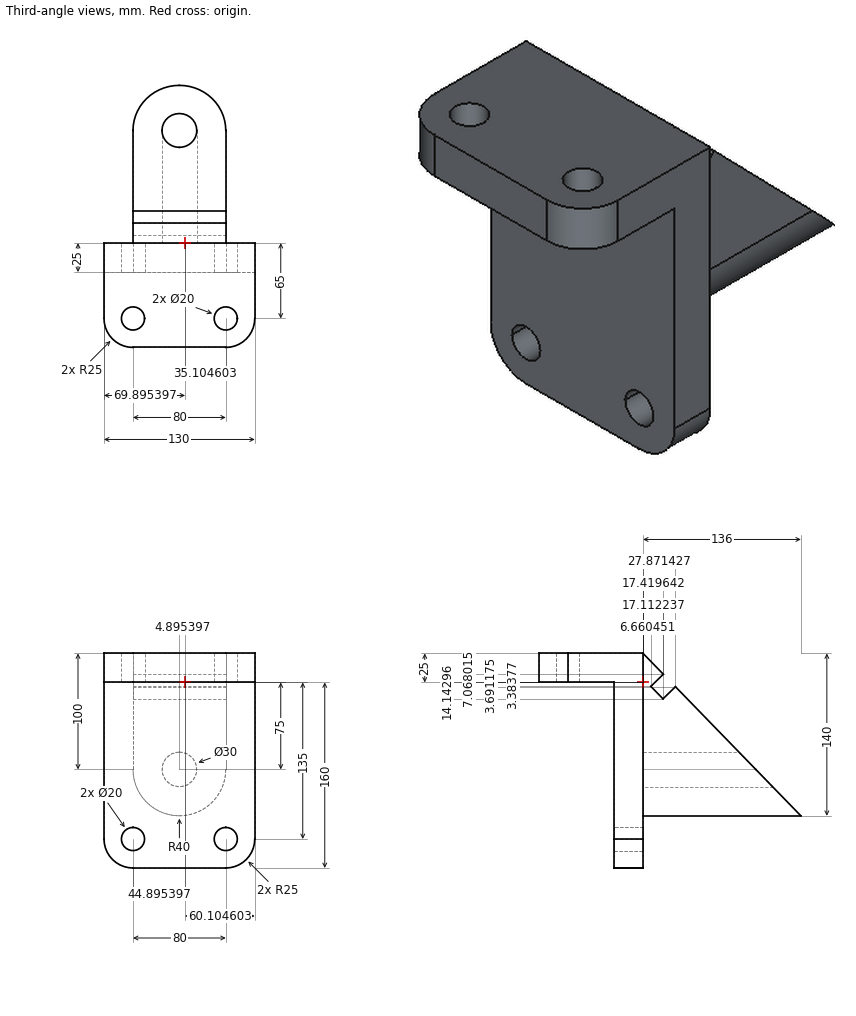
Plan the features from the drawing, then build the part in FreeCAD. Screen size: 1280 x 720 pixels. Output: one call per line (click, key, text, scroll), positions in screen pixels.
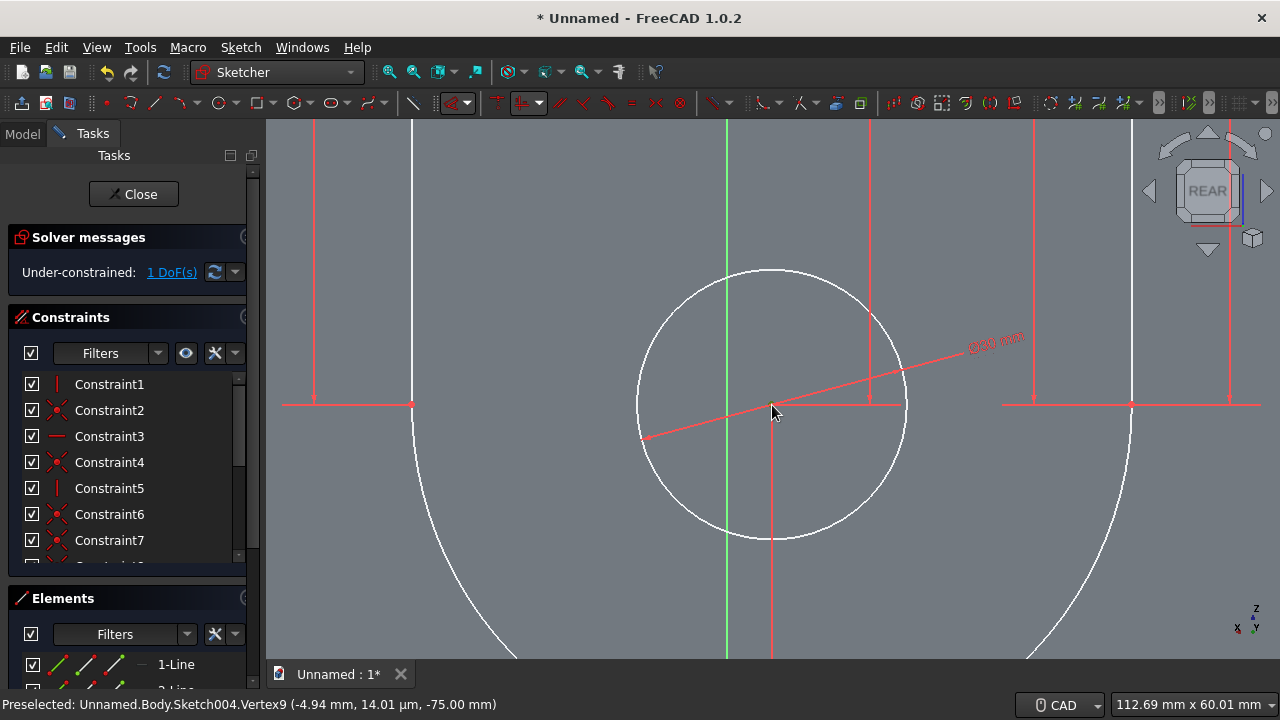
click(470, 104)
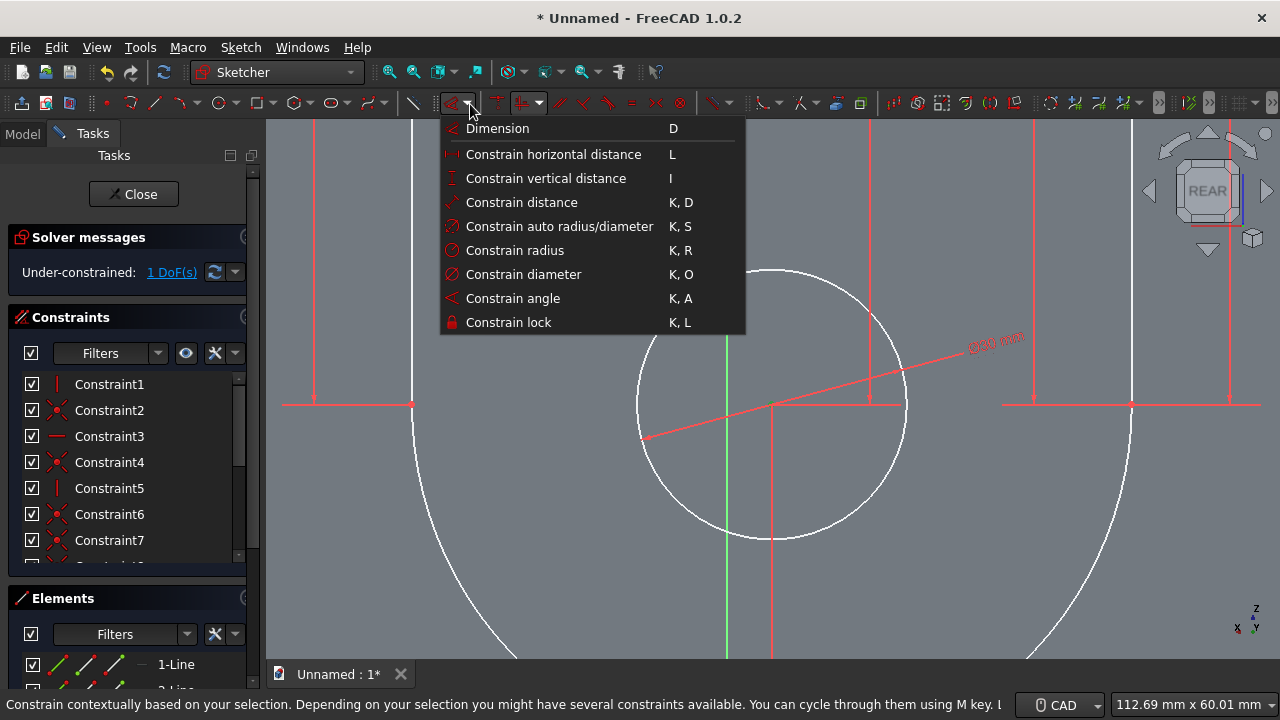
click(593, 154)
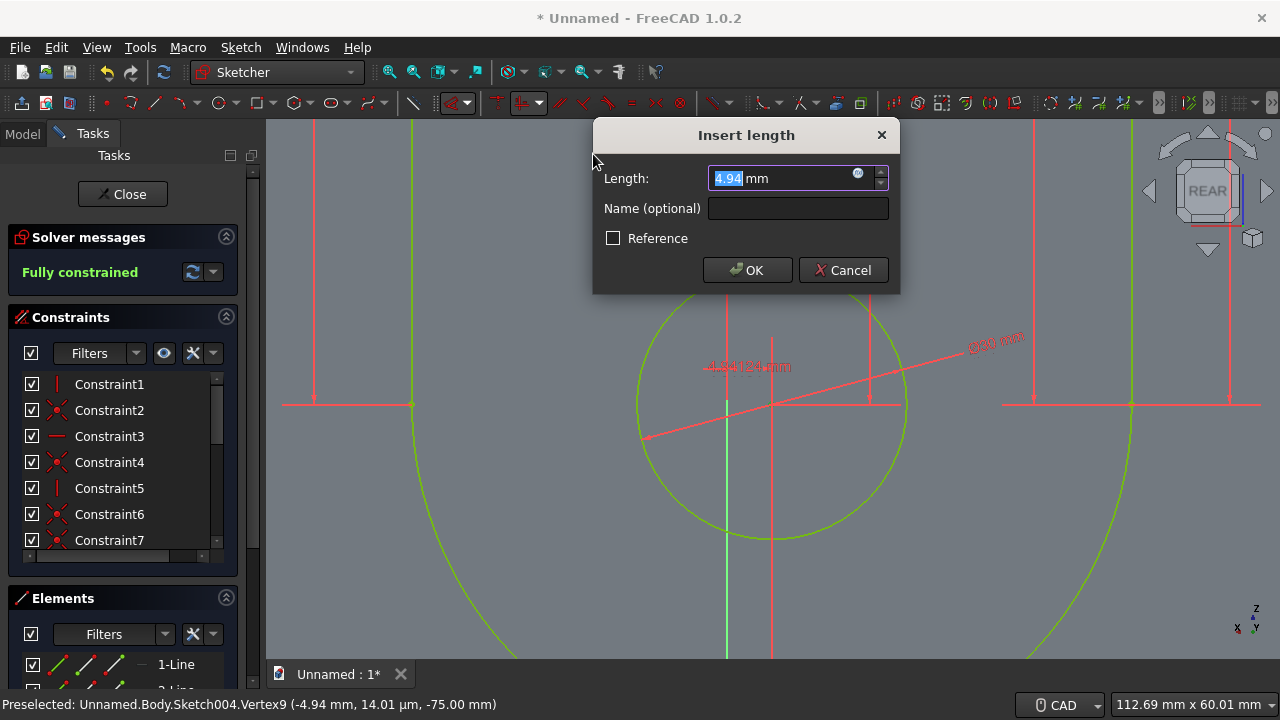
text(4.895397)
key(Return)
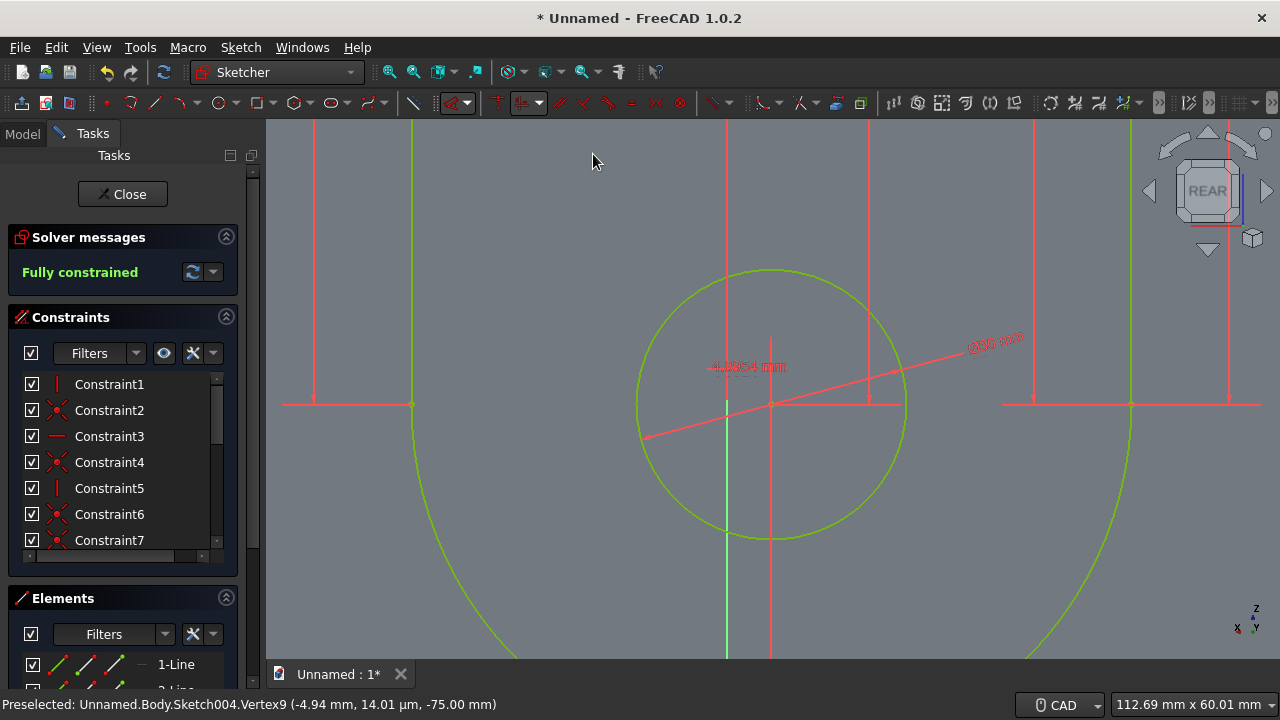
click(123, 194)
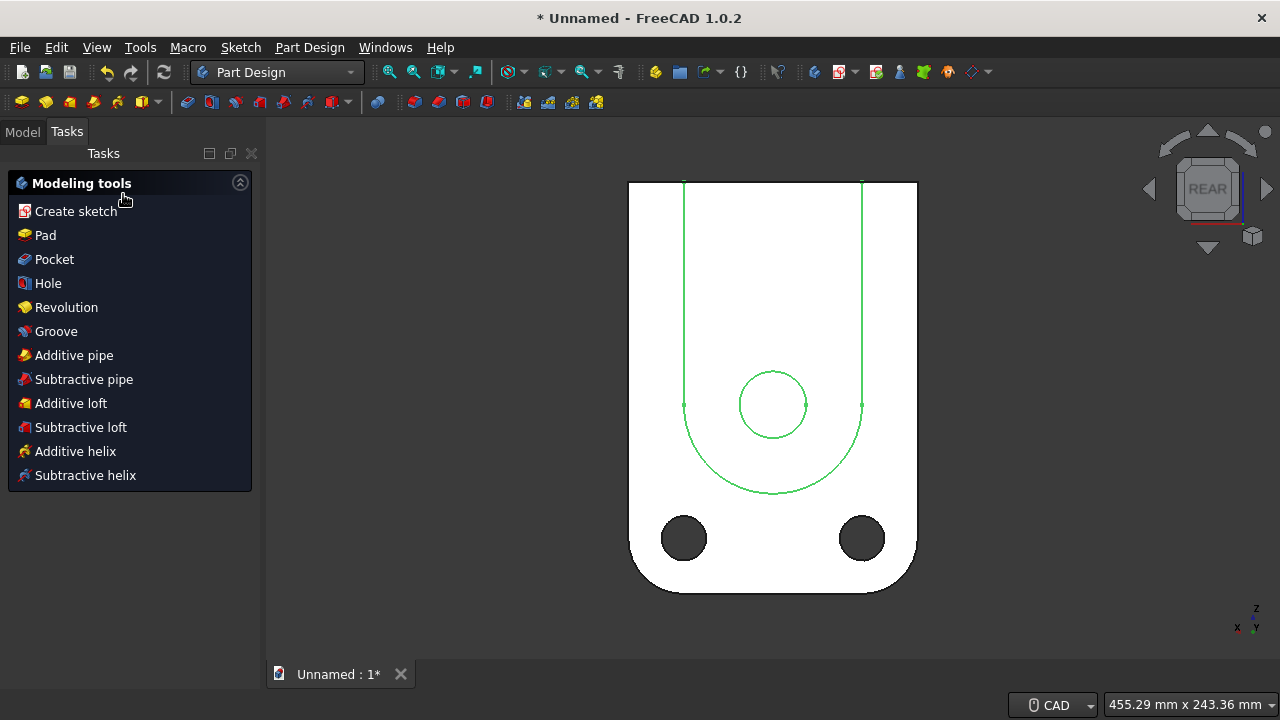
click(22, 102)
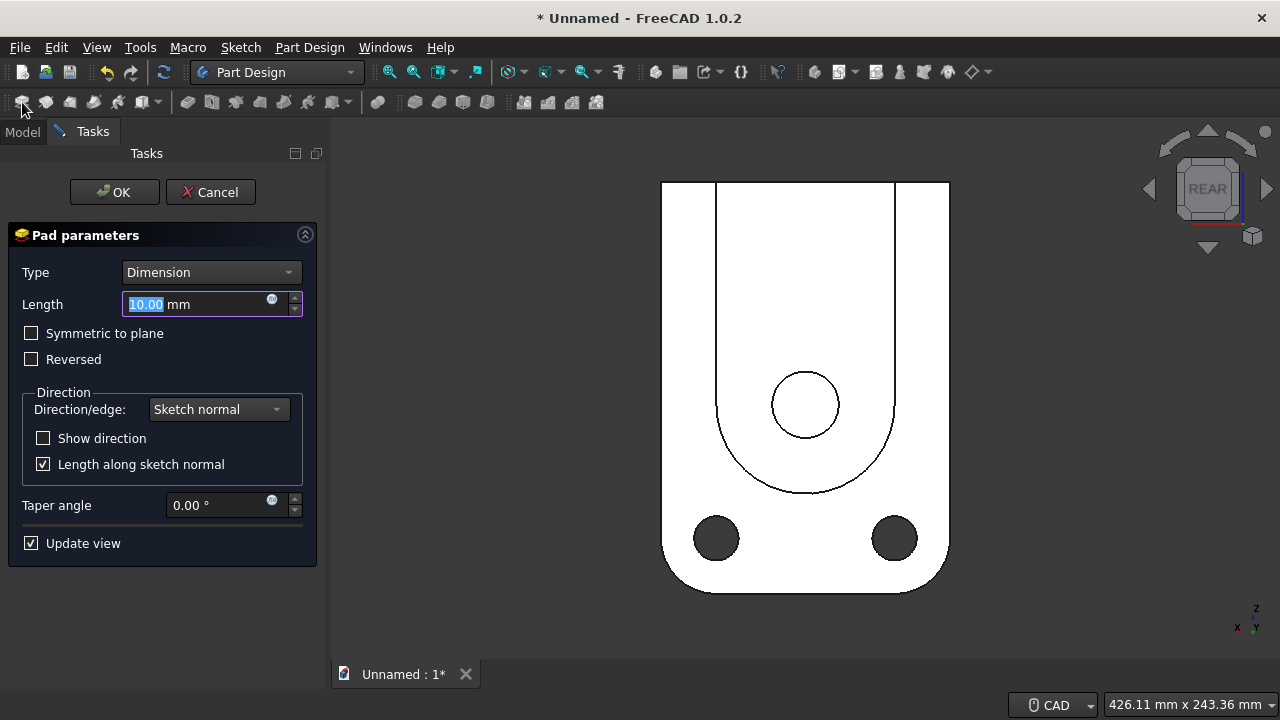
text(136)
key(Tab)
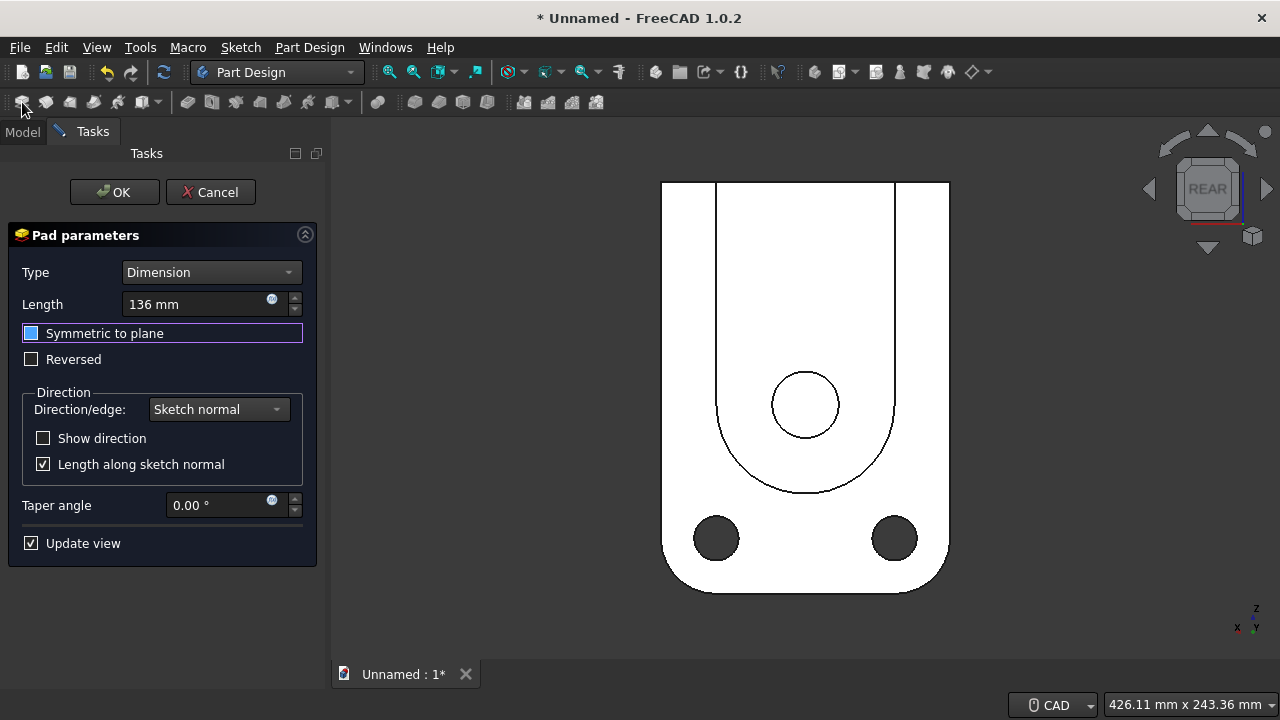
click(115, 192)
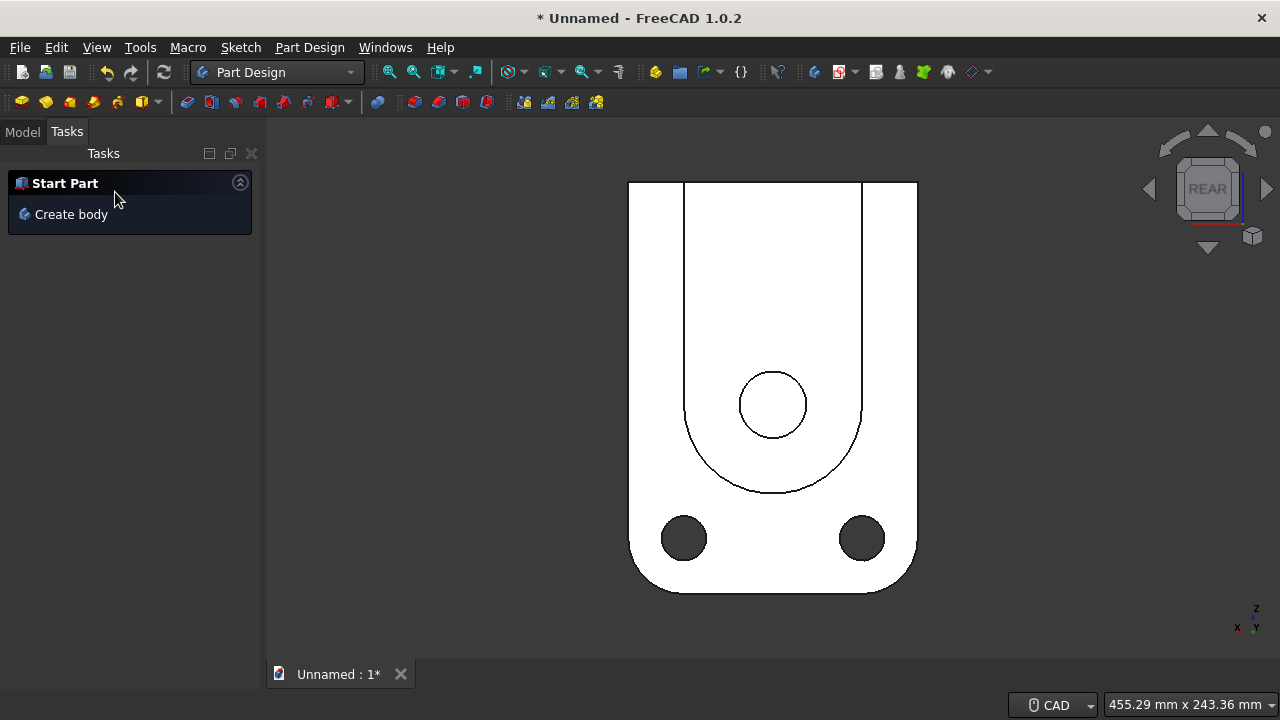
key(0)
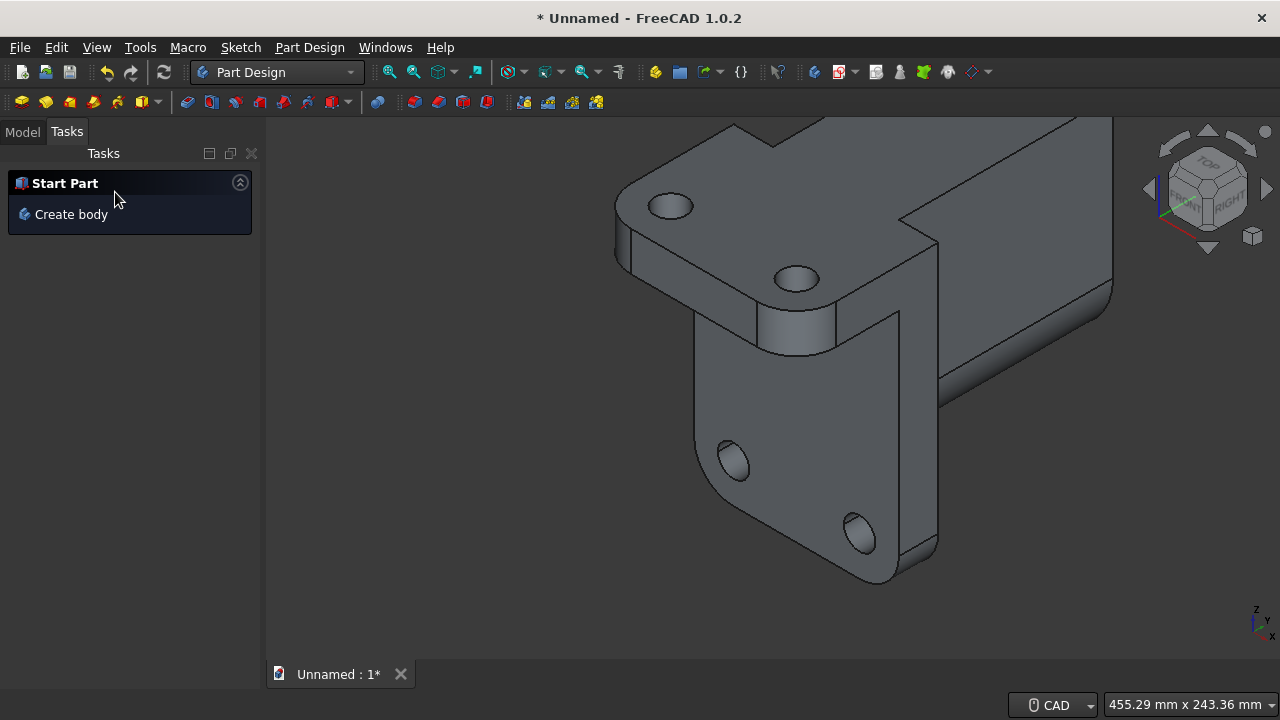
click(390, 72)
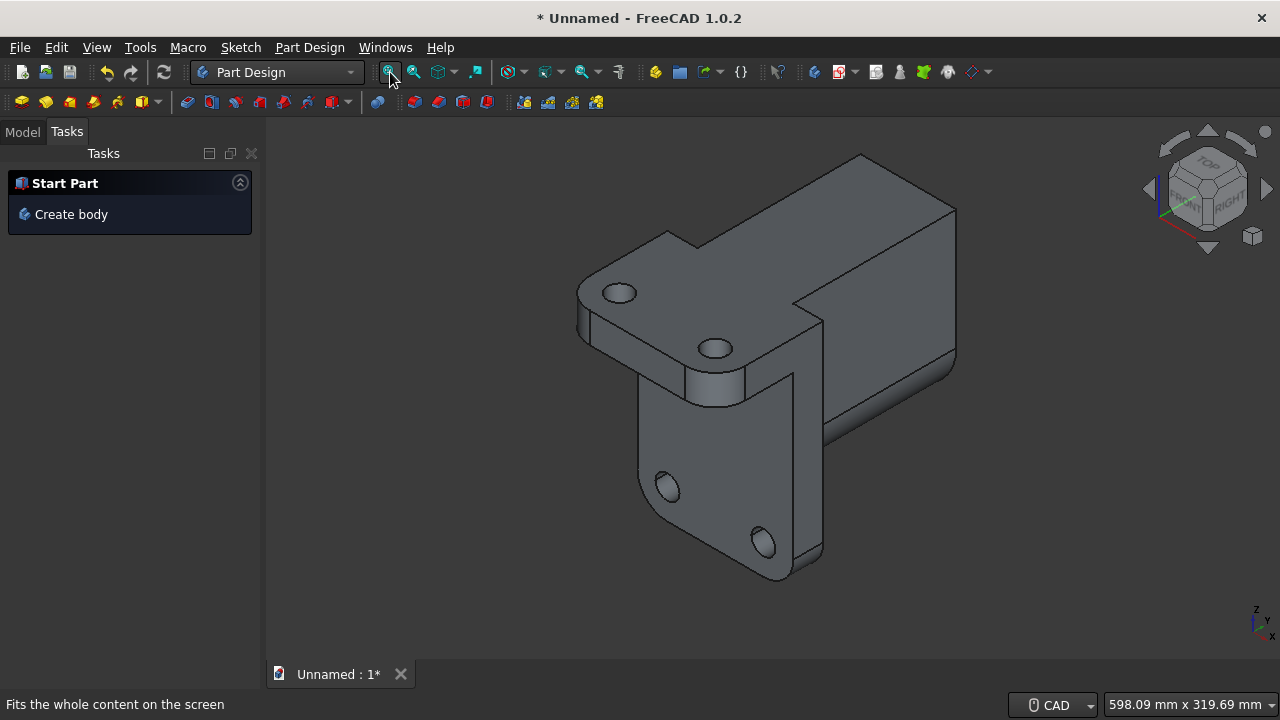
click(875, 325)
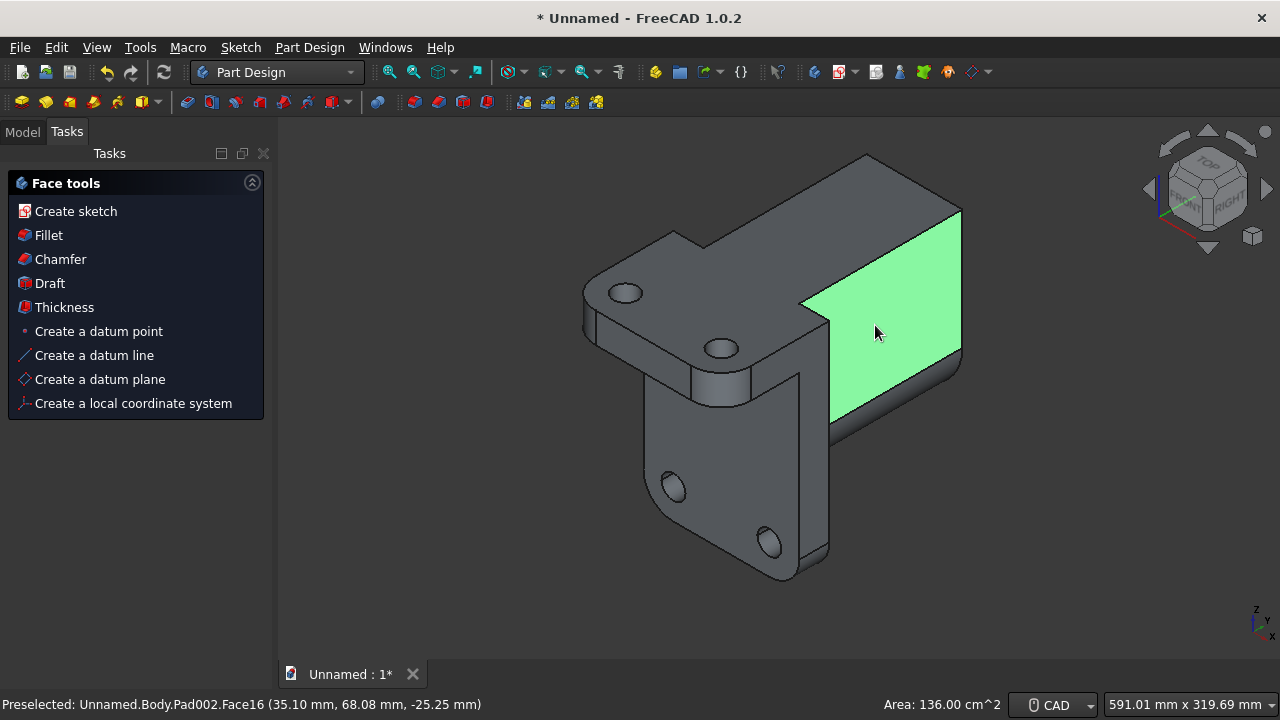
click(840, 72)